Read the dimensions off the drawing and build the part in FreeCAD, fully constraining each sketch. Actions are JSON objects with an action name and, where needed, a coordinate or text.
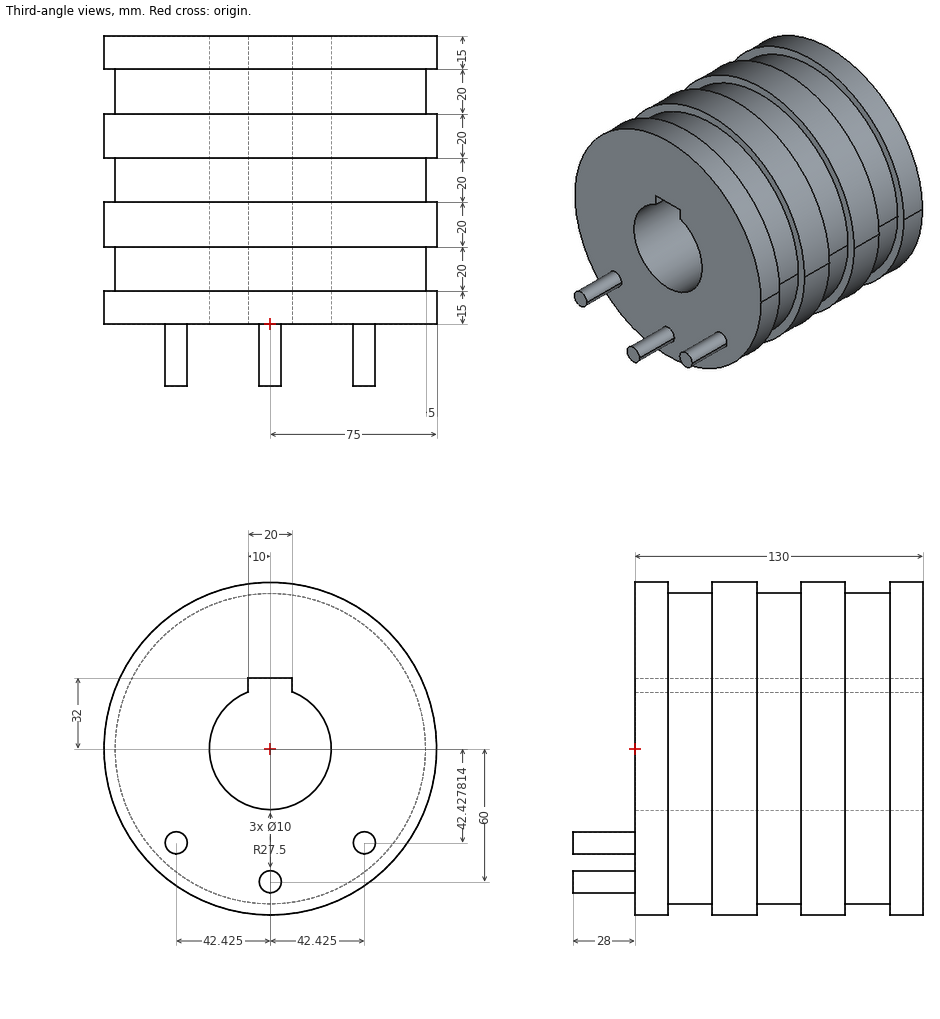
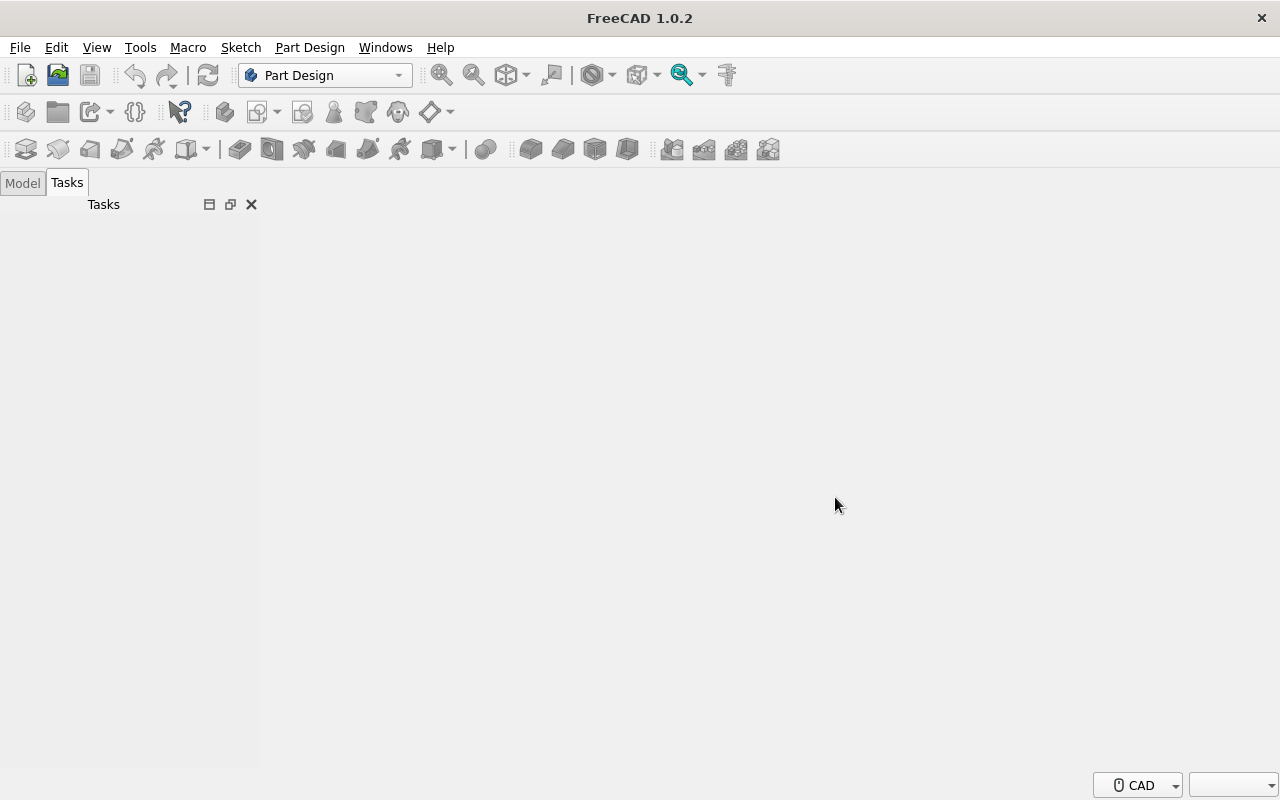
{"action": "key", "text": "ctrl+n"}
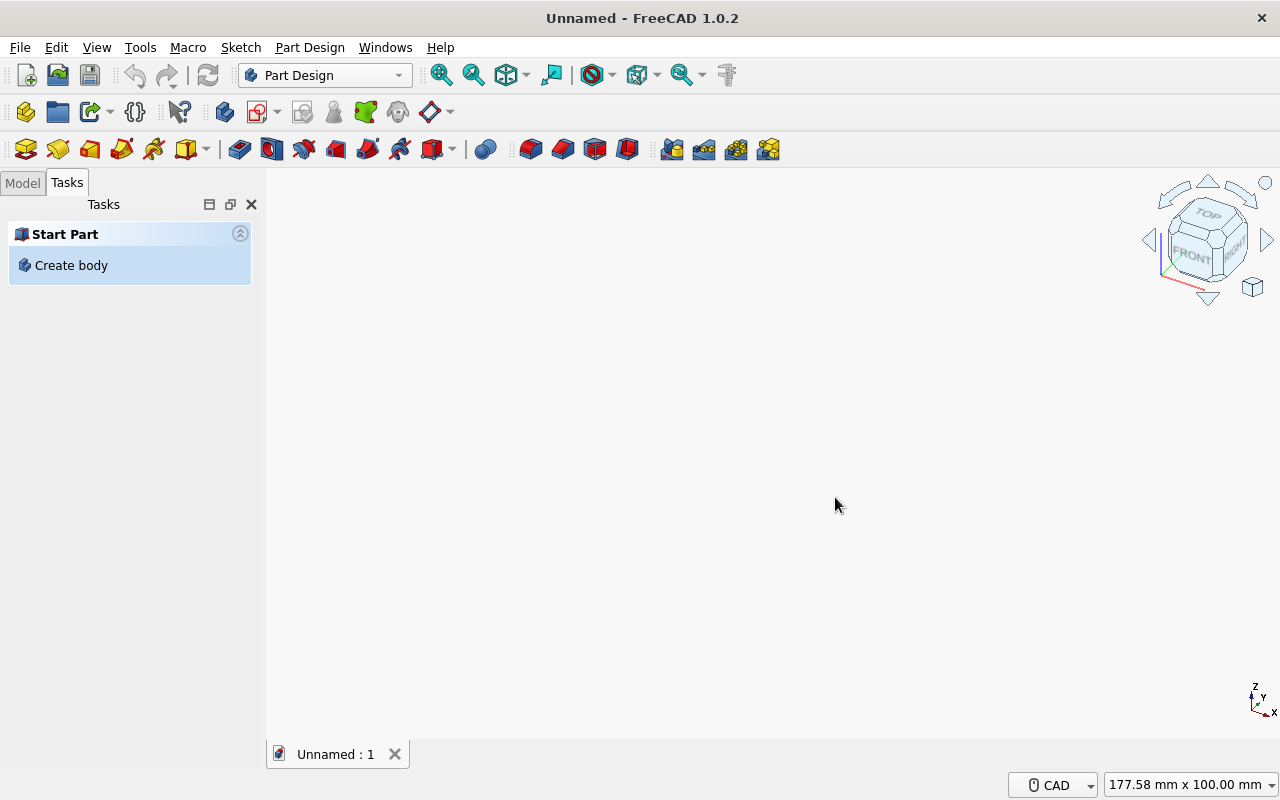
{"action": "left_click", "coordinate": [258, 112]}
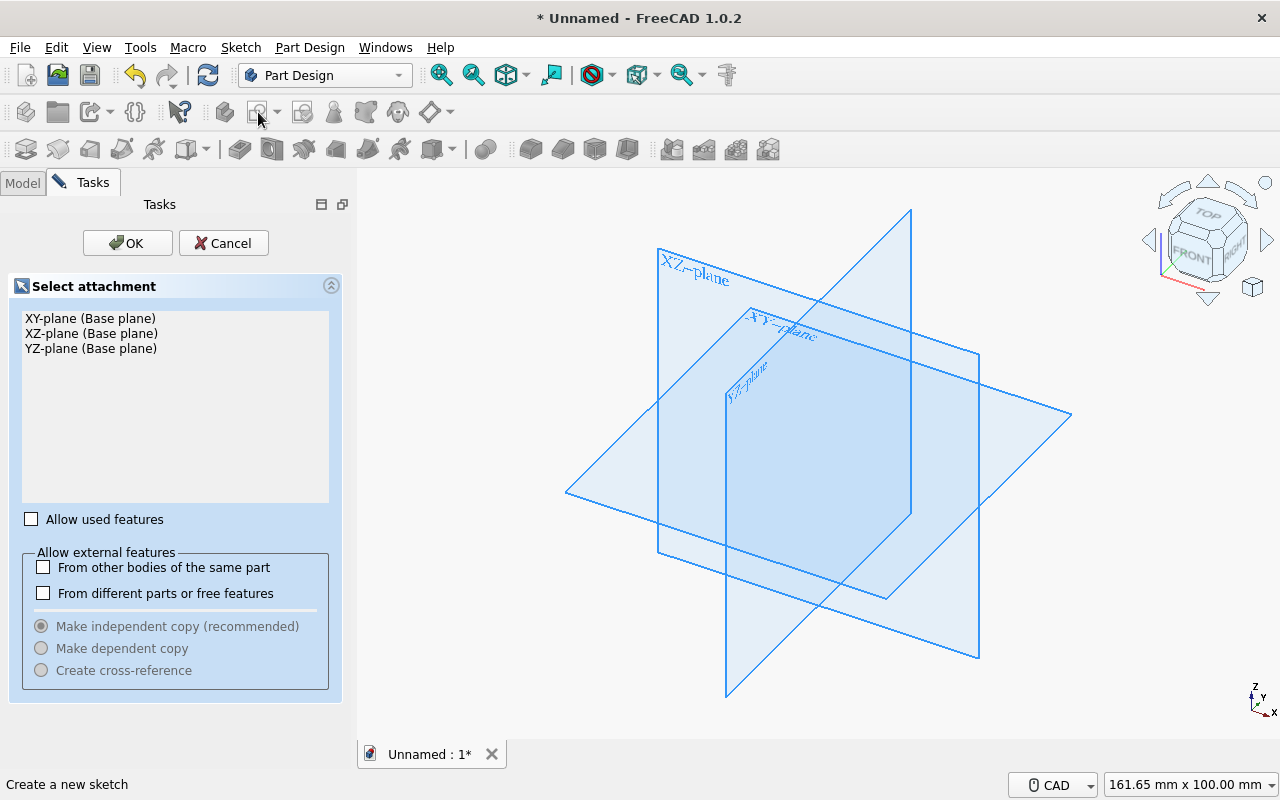
{"action": "left_click", "coordinate": [82, 318]}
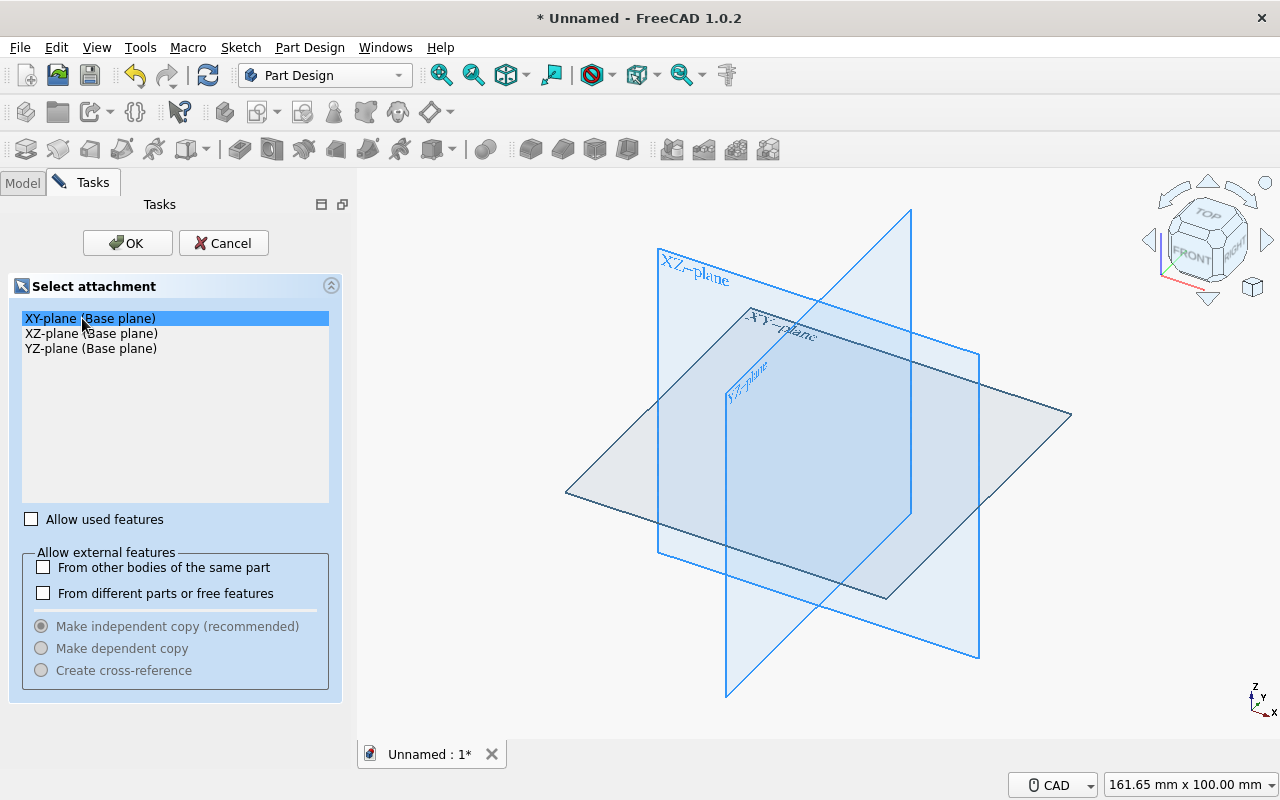
{"action": "left_click", "coordinate": [128, 243]}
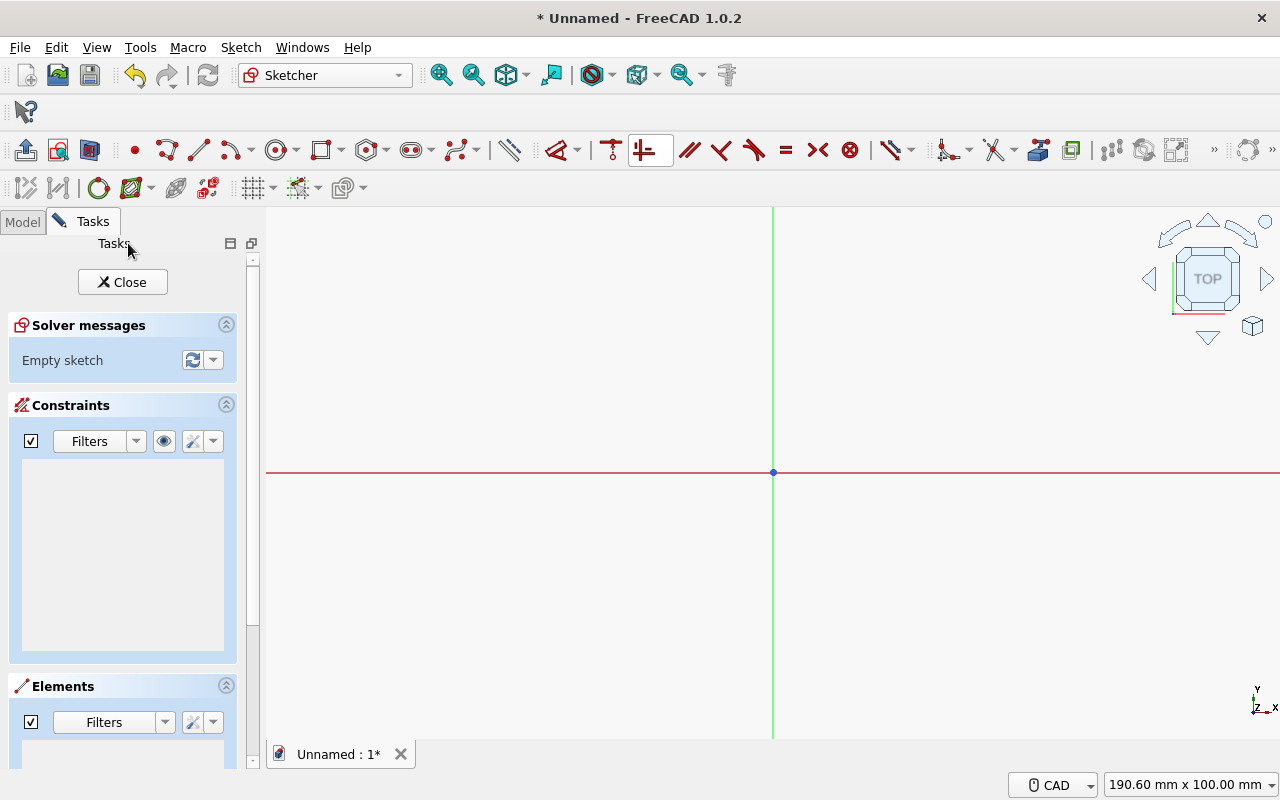
{"action": "scroll", "coordinate": [486, 711], "scroll_direction": "down", "scroll_amount": 4}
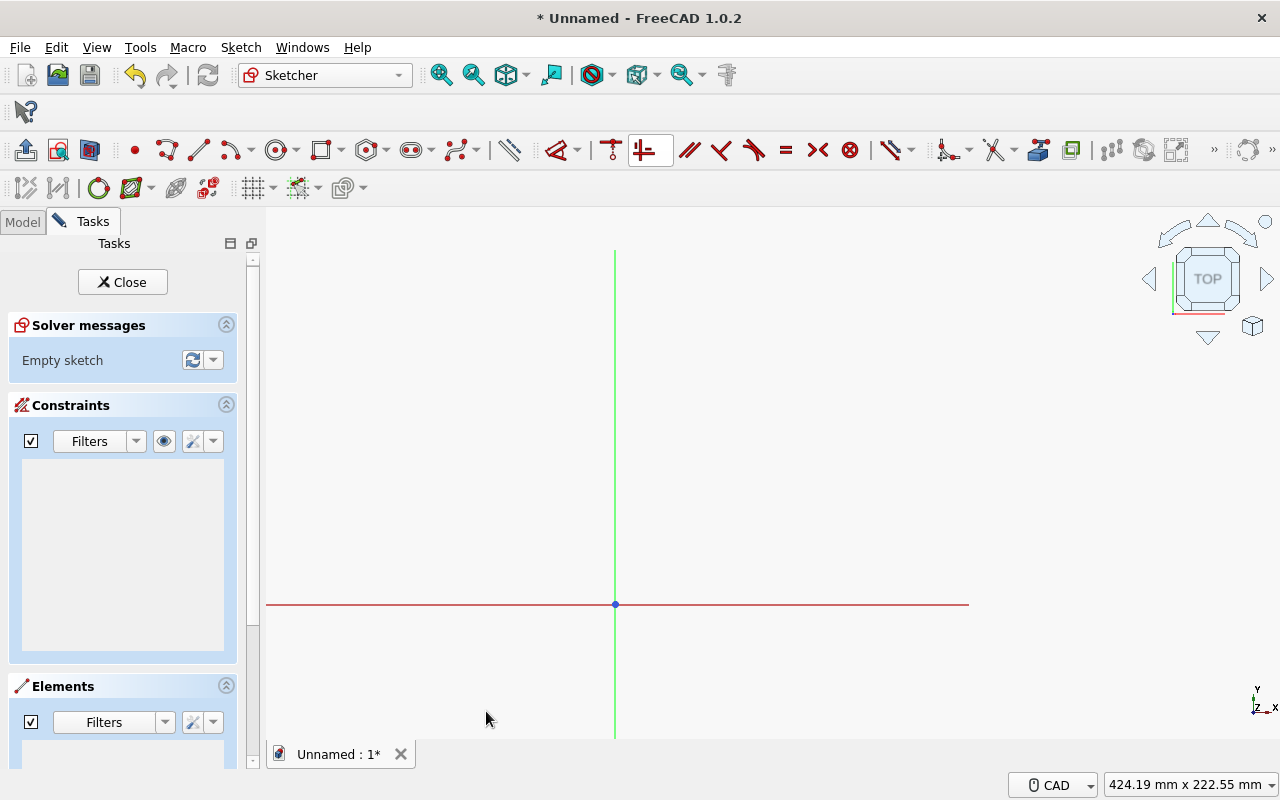
{"action": "left_click", "coordinate": [168, 150]}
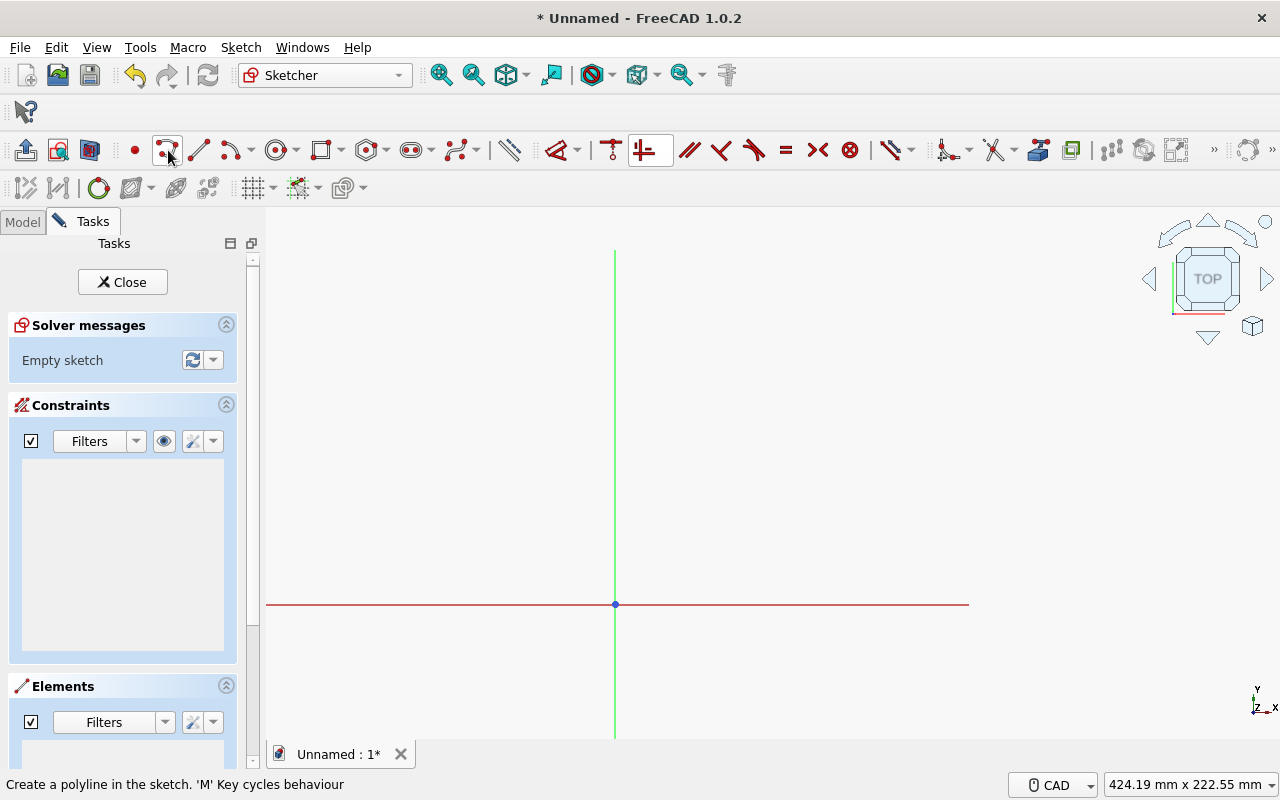
{"action": "left_click", "coordinate": [615, 605]}
{"action": "left_click", "coordinate": [794, 596]}
{"action": "left_click", "coordinate": [794, 569]}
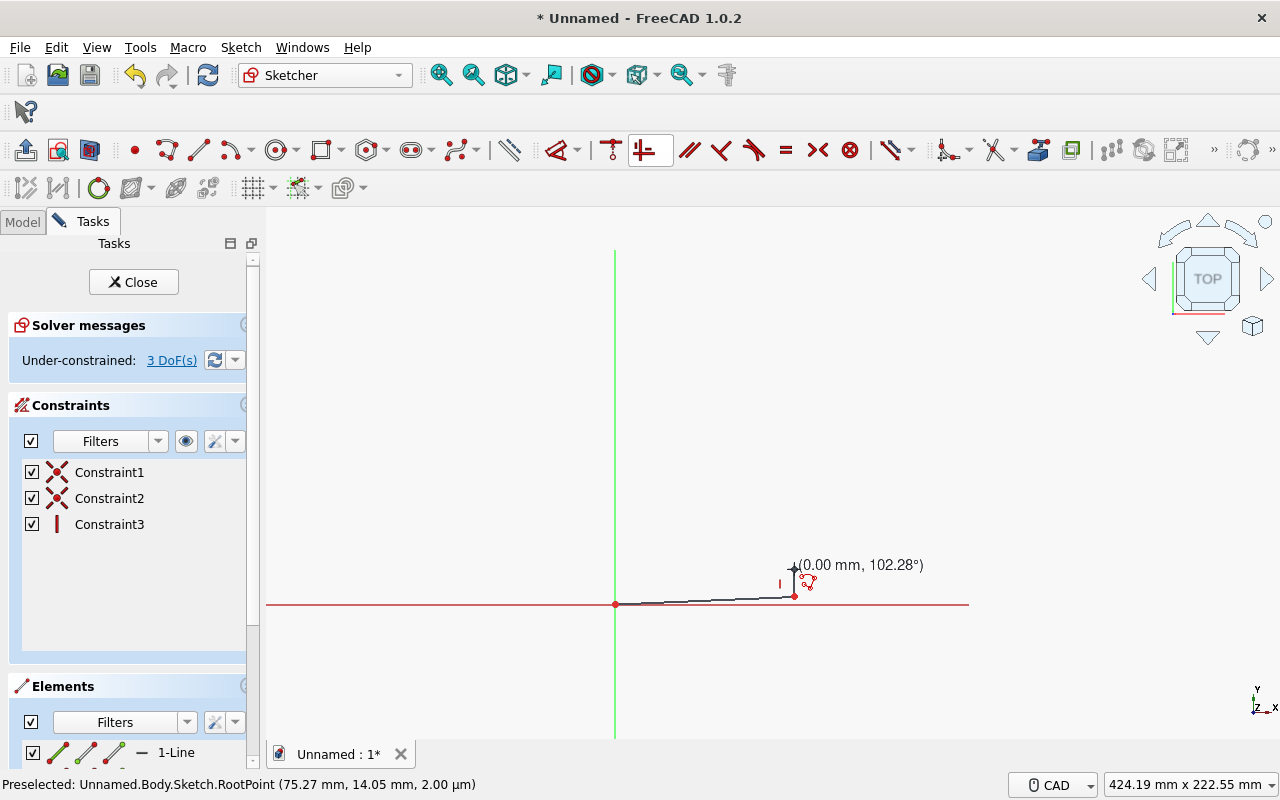
{"action": "scroll", "coordinate": [782, 569], "scroll_direction": "up", "scroll_amount": 2}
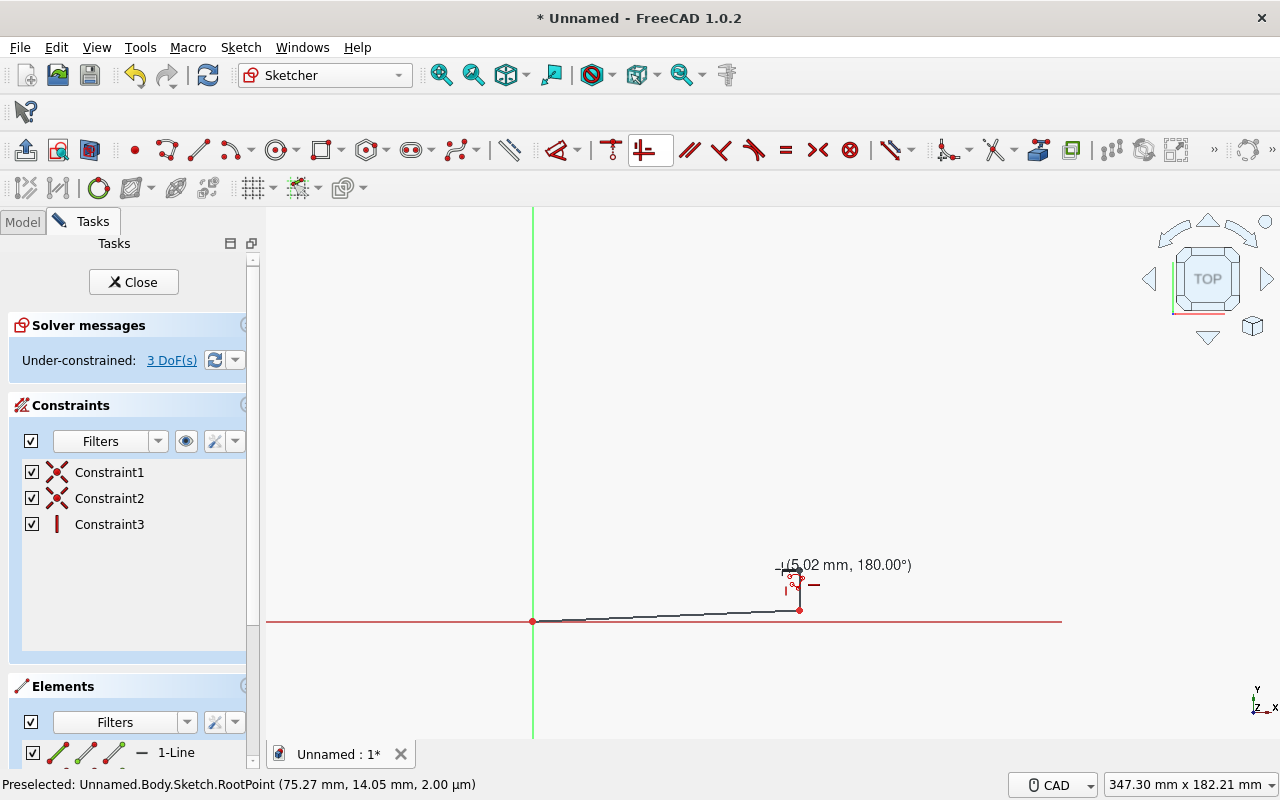
{"action": "left_click", "coordinate": [782, 569]}
{"action": "left_click", "coordinate": [782, 497]}
{"action": "left_click", "coordinate": [800, 497]}
{"action": "left_click", "coordinate": [800, 426]}
{"action": "left_click", "coordinate": [782, 426]}
{"action": "left_click", "coordinate": [782, 354]}
{"action": "left_click", "coordinate": [800, 354]}
{"action": "left_click", "coordinate": [800, 283]}
{"action": "left_click", "coordinate": [782, 283]}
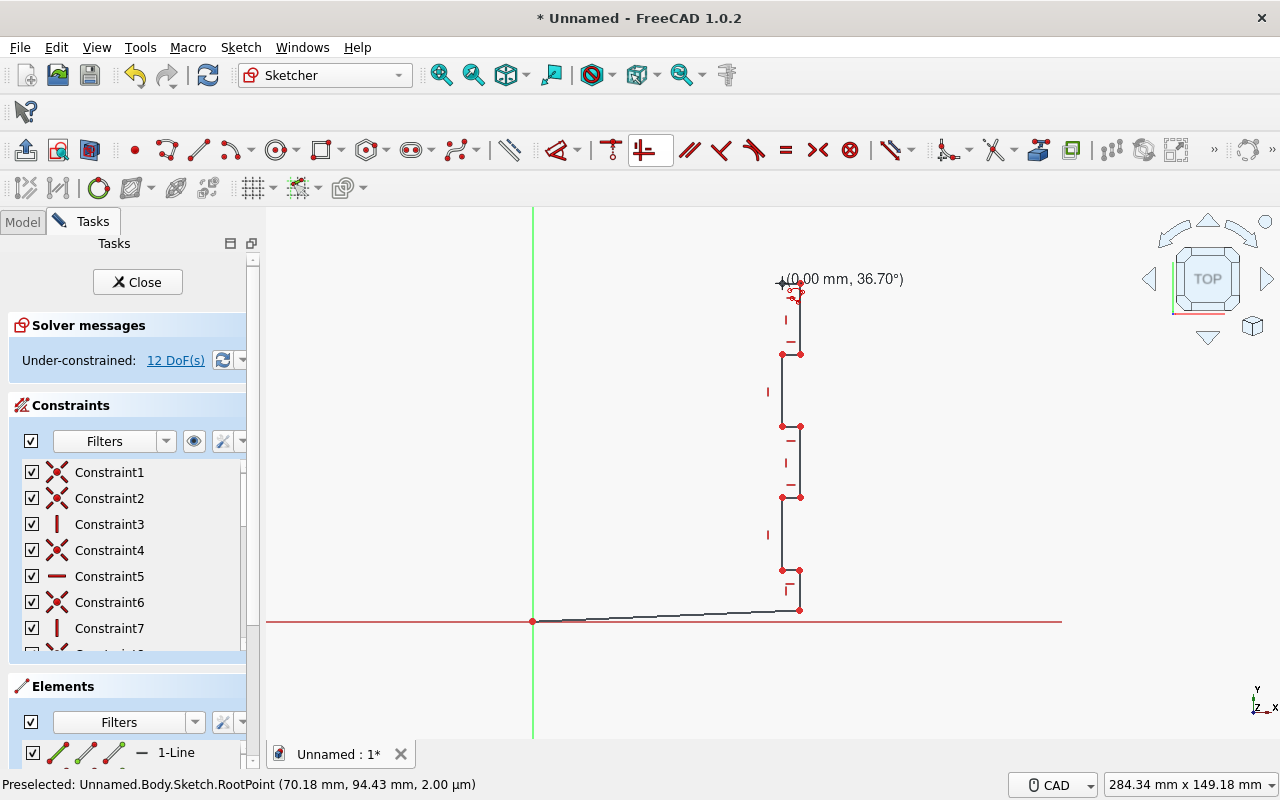
{"action": "scroll", "coordinate": [782, 642], "scroll_direction": "down", "scroll_amount": 2}